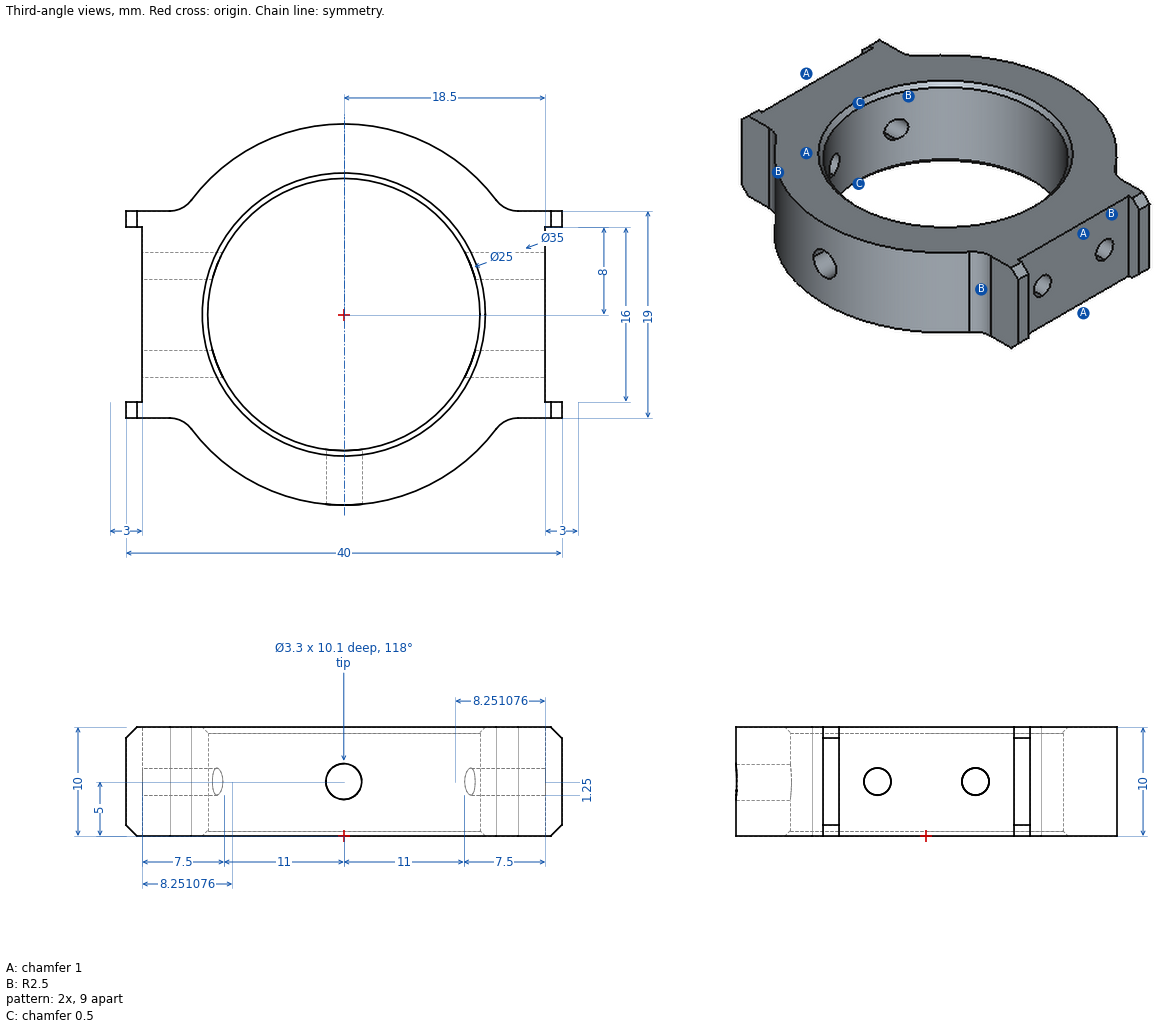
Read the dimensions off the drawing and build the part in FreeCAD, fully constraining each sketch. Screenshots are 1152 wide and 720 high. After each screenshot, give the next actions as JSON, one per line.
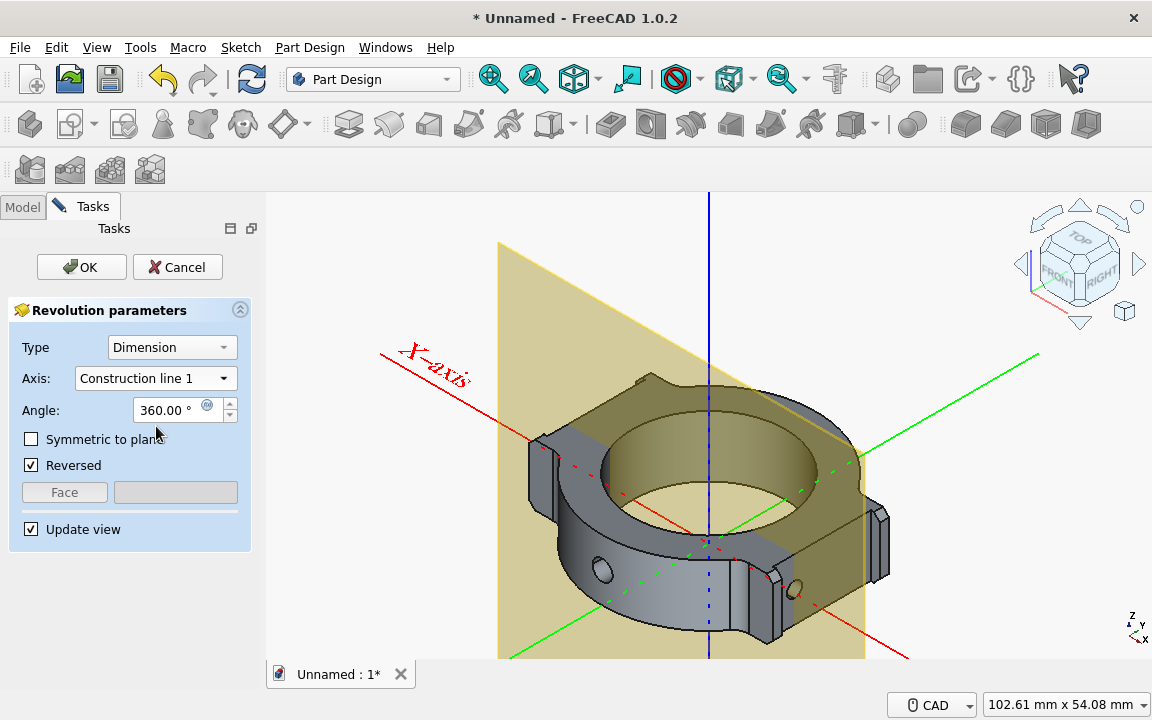
{"action": "left_click", "coordinate": [82, 267]}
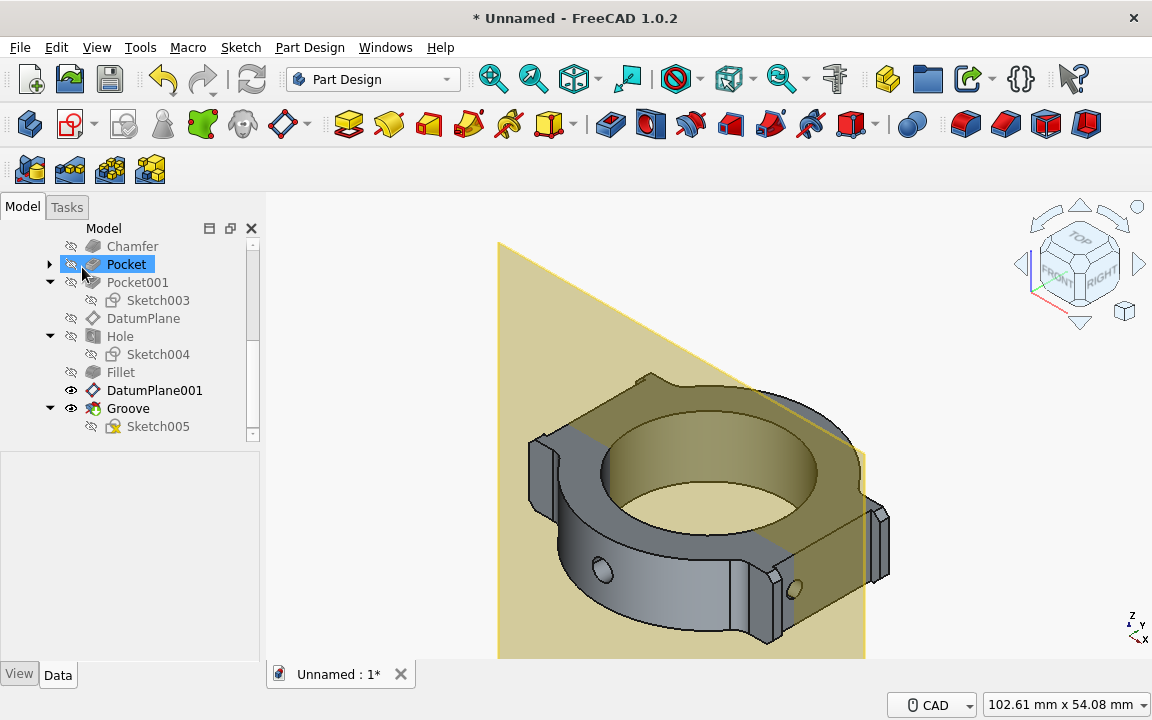
{"action": "left_click", "coordinate": [116, 390]}
{"action": "key", "text": "space"}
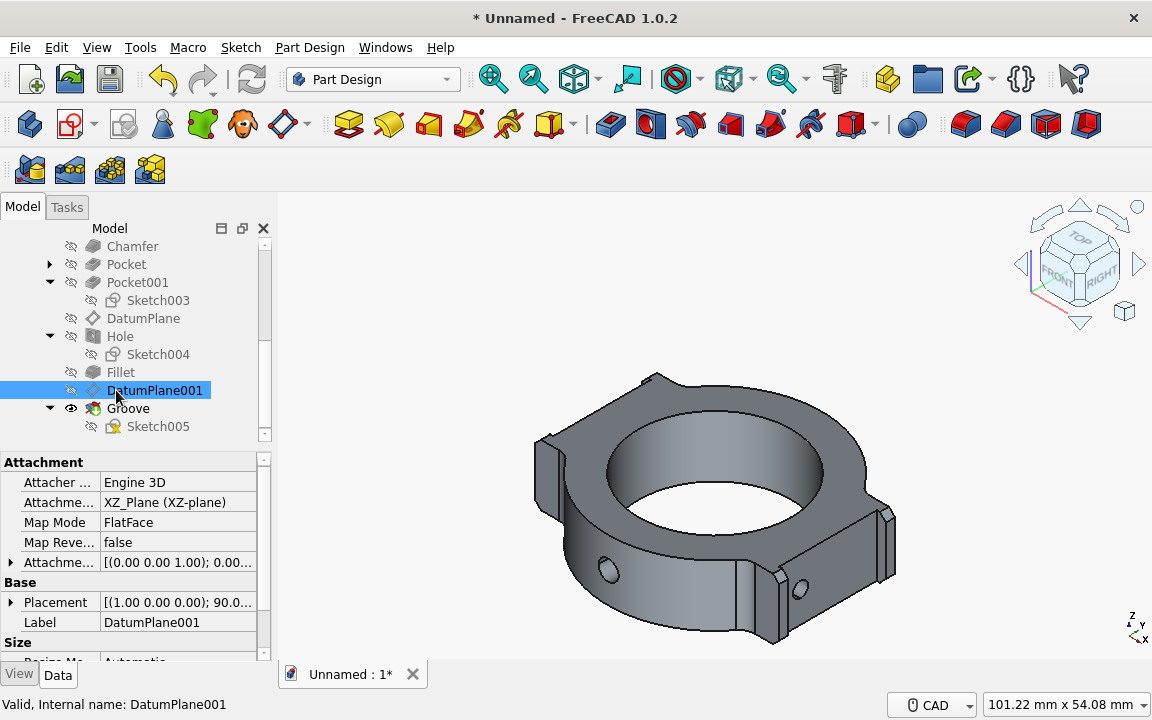
{"action": "left_click", "coordinate": [494, 80]}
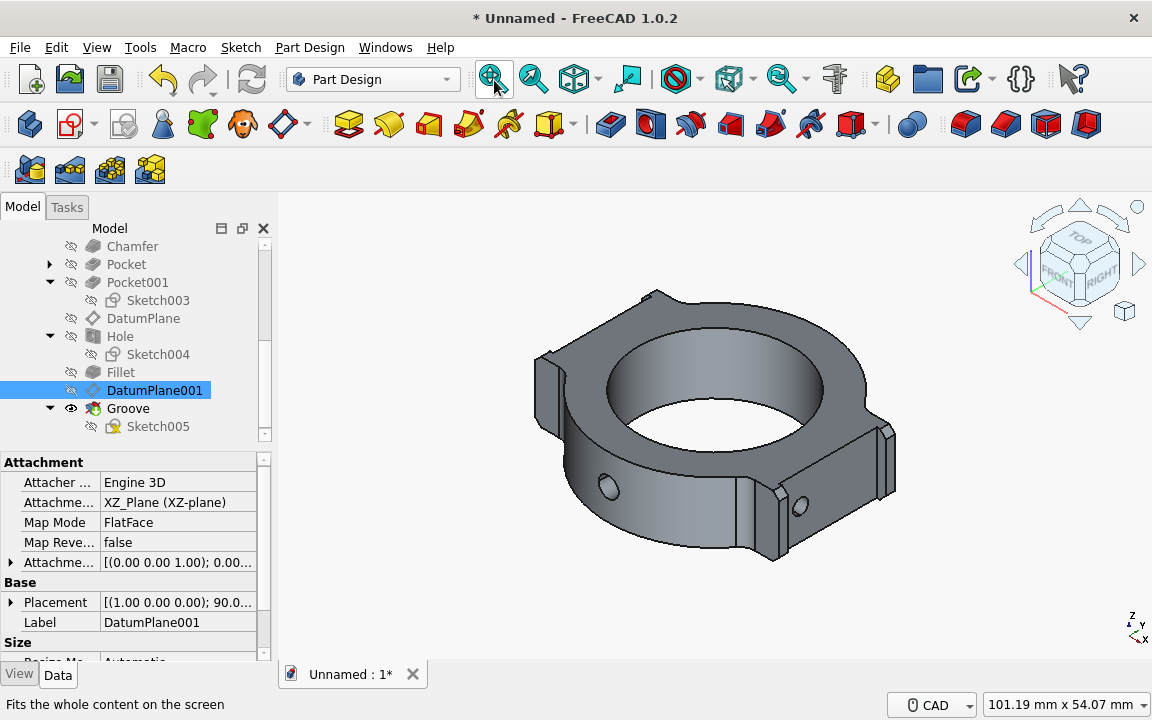
{"action": "left_click", "coordinate": [116, 408]}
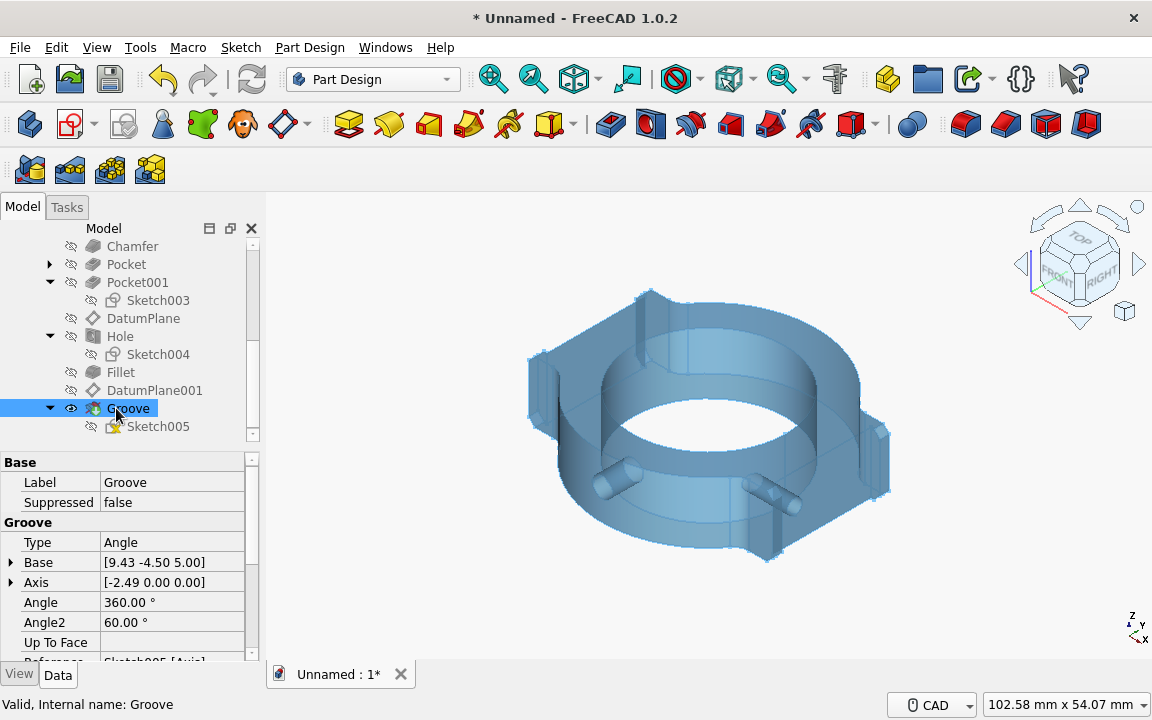
{"action": "left_click", "coordinate": [70, 170]}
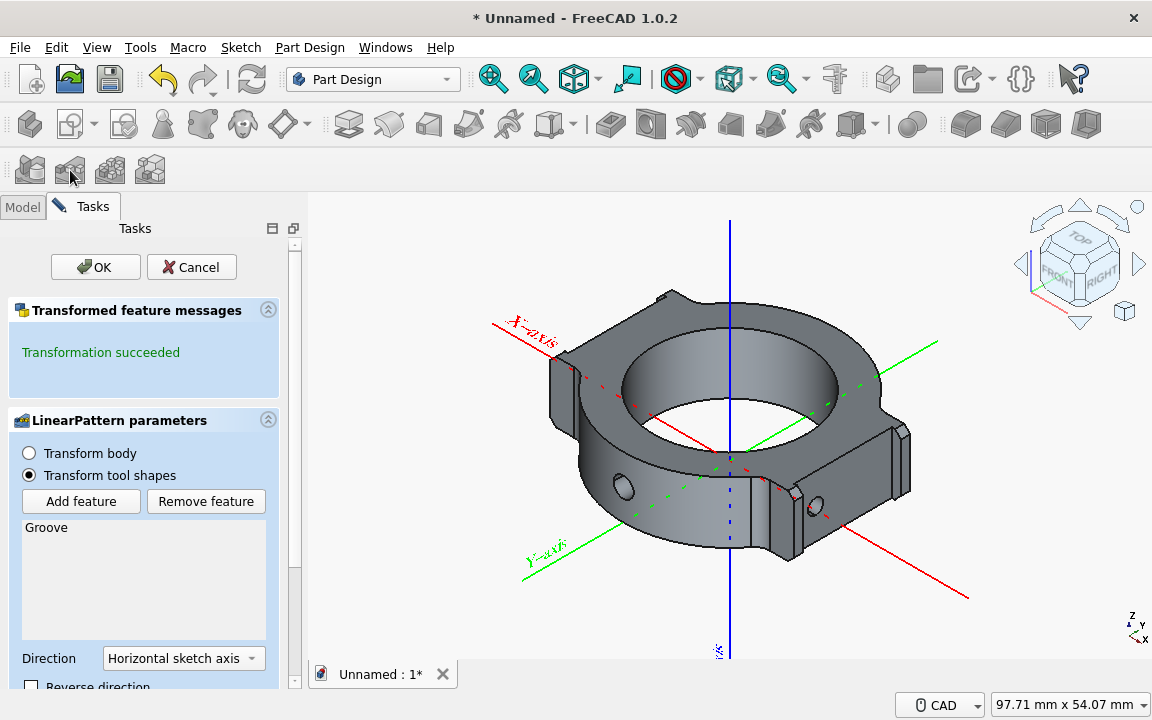
{"action": "left_click", "coordinate": [184, 658]}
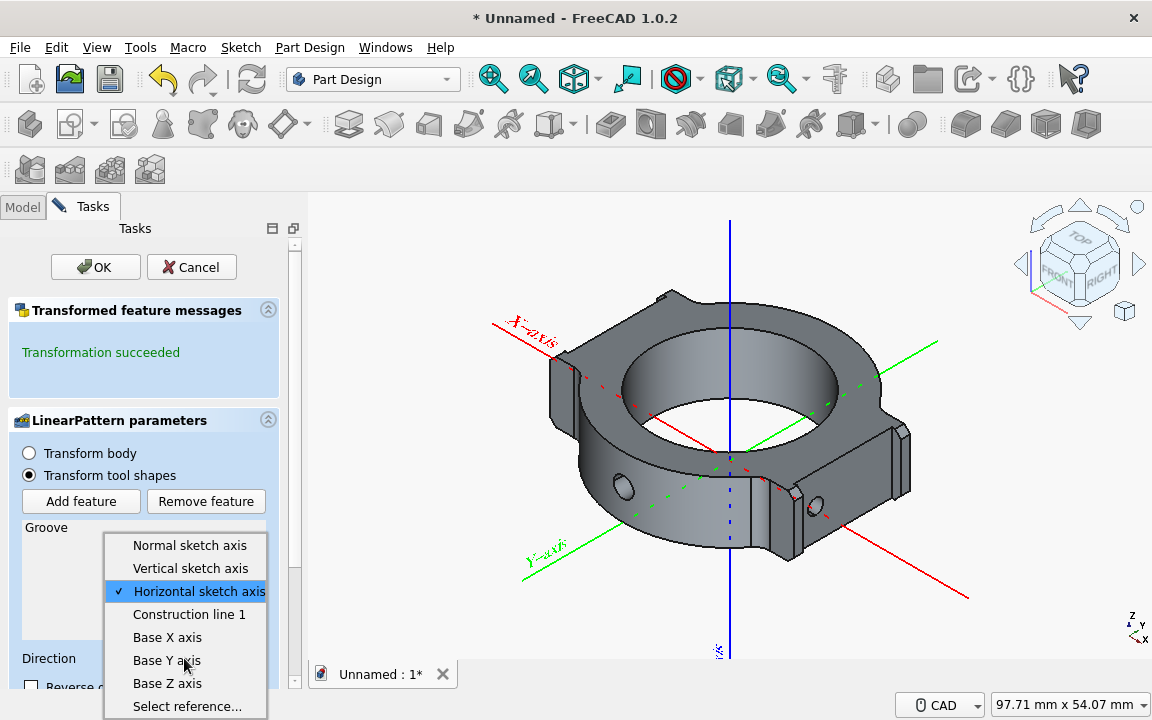
{"action": "left_click", "coordinate": [184, 660]}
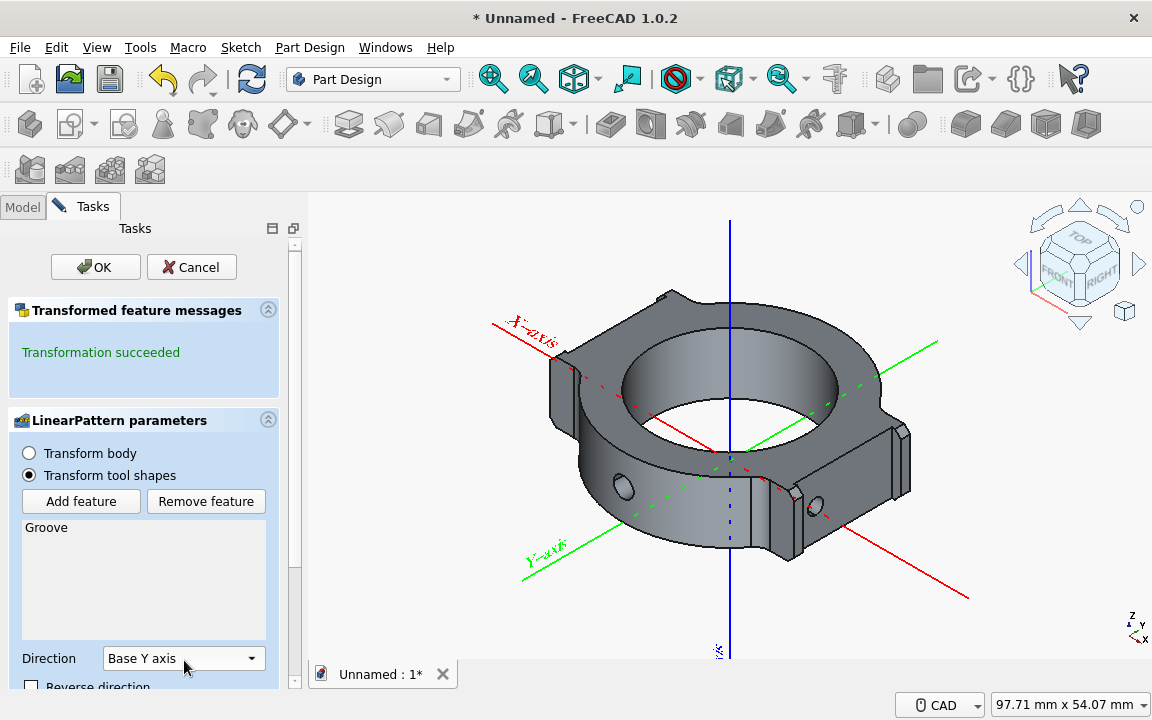
{"action": "scroll", "coordinate": [295, 463], "scroll_direction": "down", "scroll_amount": 2}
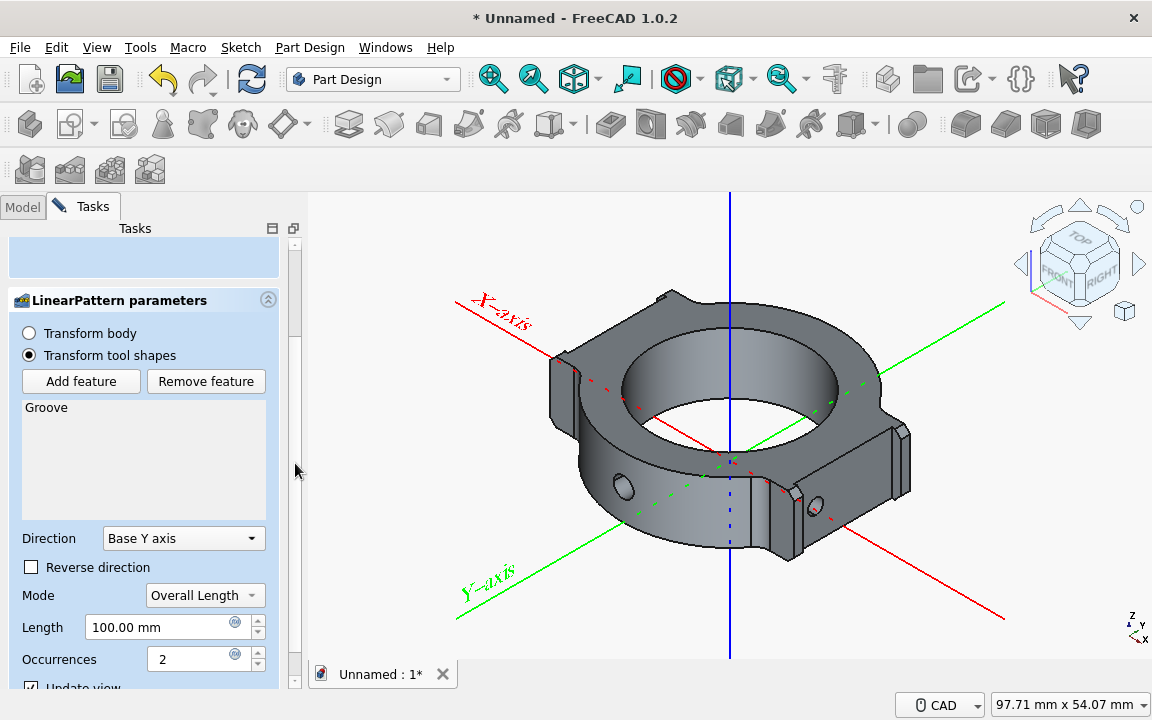
{"action": "left_click", "coordinate": [206, 596]}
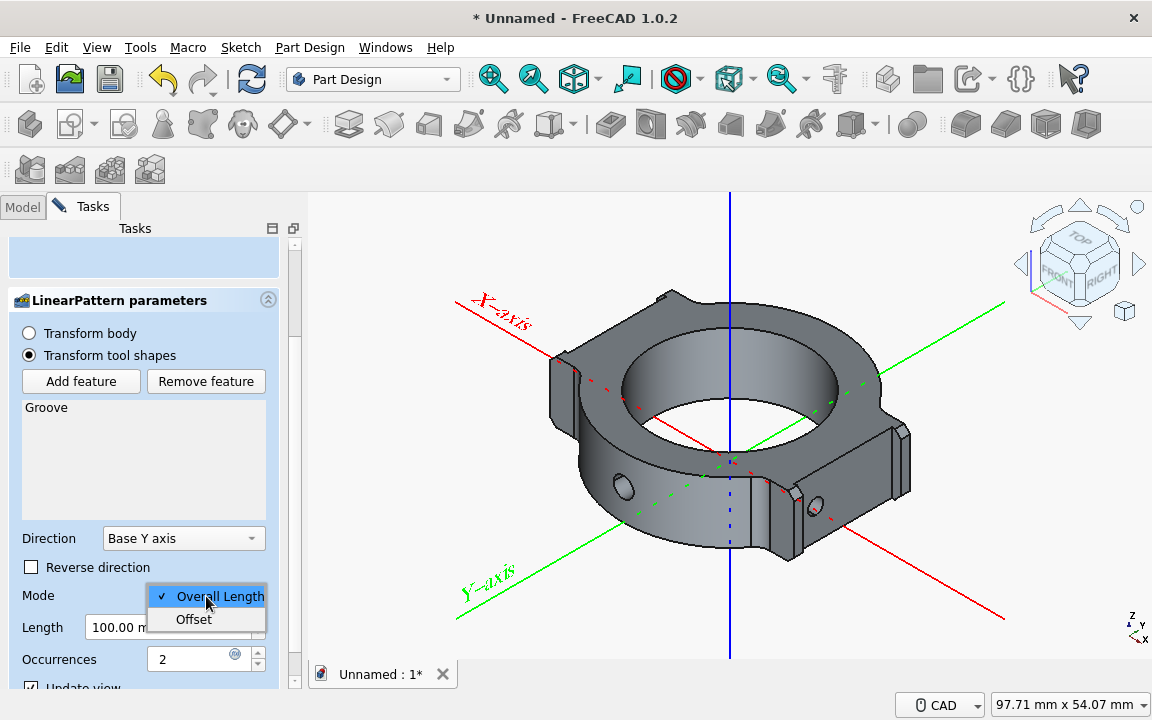
{"action": "left_click", "coordinate": [206, 620]}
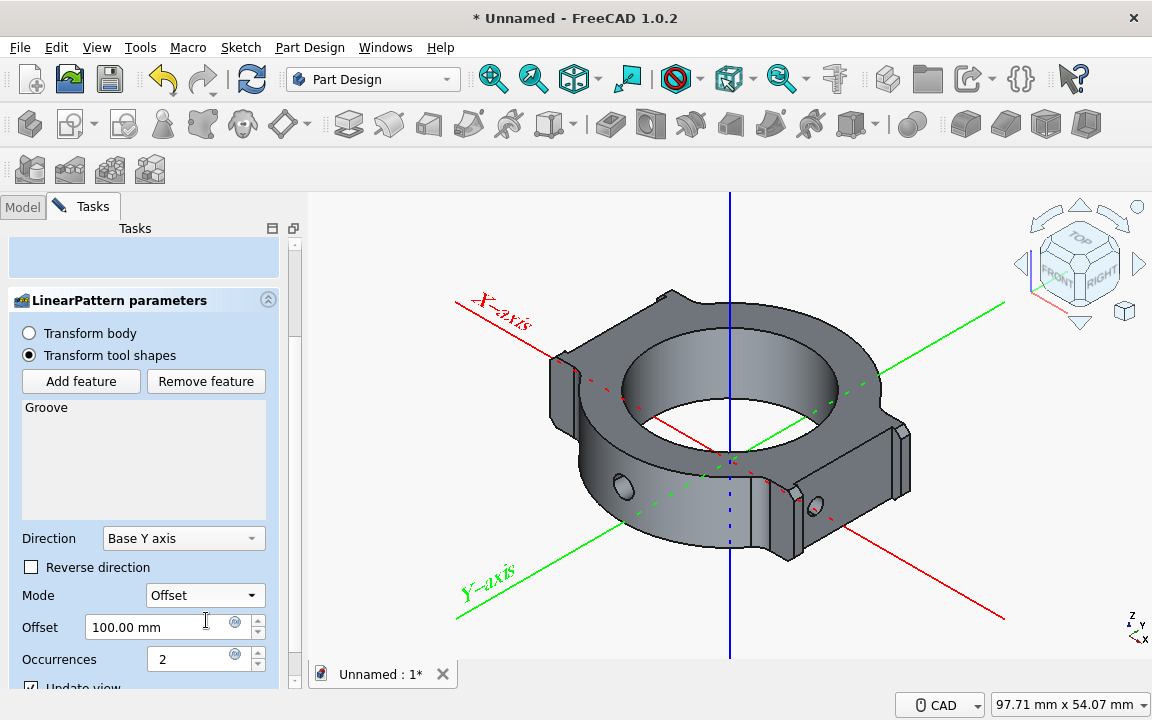
{"action": "triple_click", "coordinate": [168, 627]}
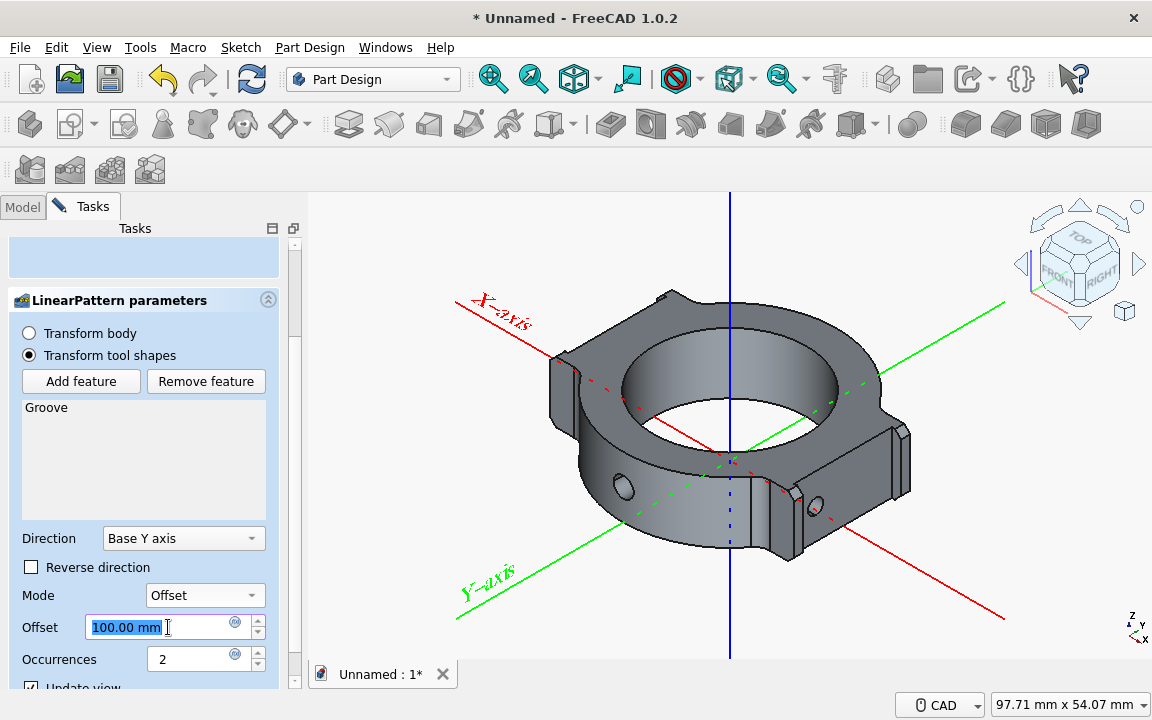
{"action": "type", "text": "9"}
{"action": "key", "text": "Tab"}